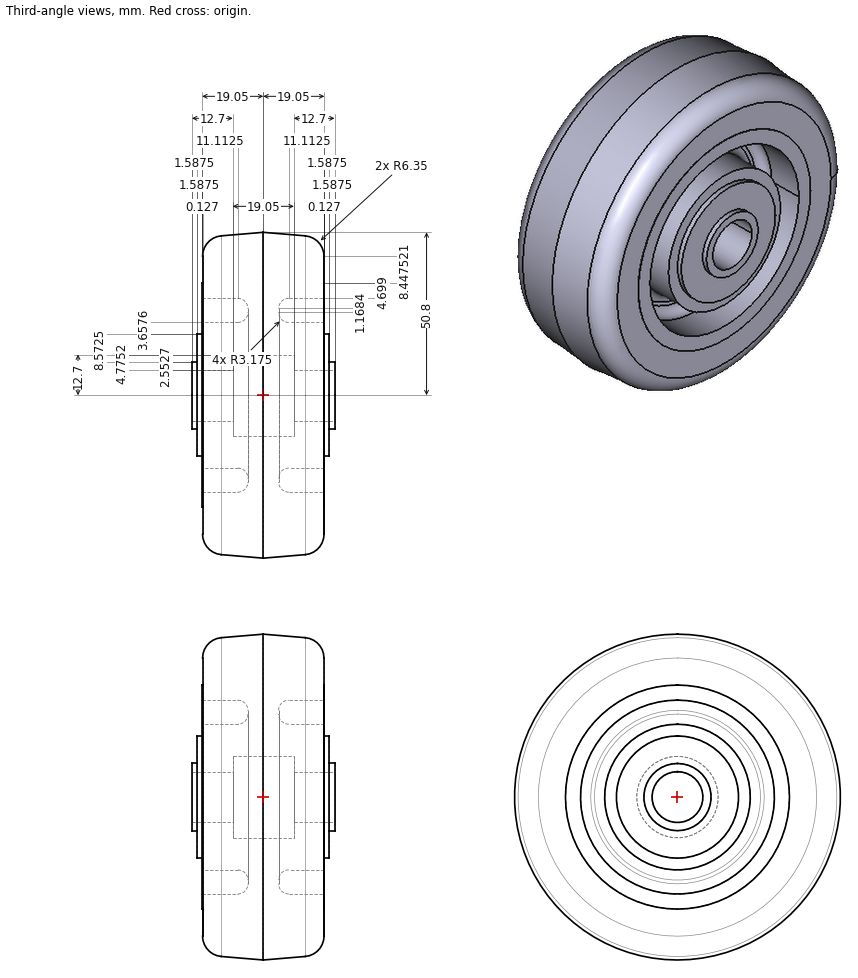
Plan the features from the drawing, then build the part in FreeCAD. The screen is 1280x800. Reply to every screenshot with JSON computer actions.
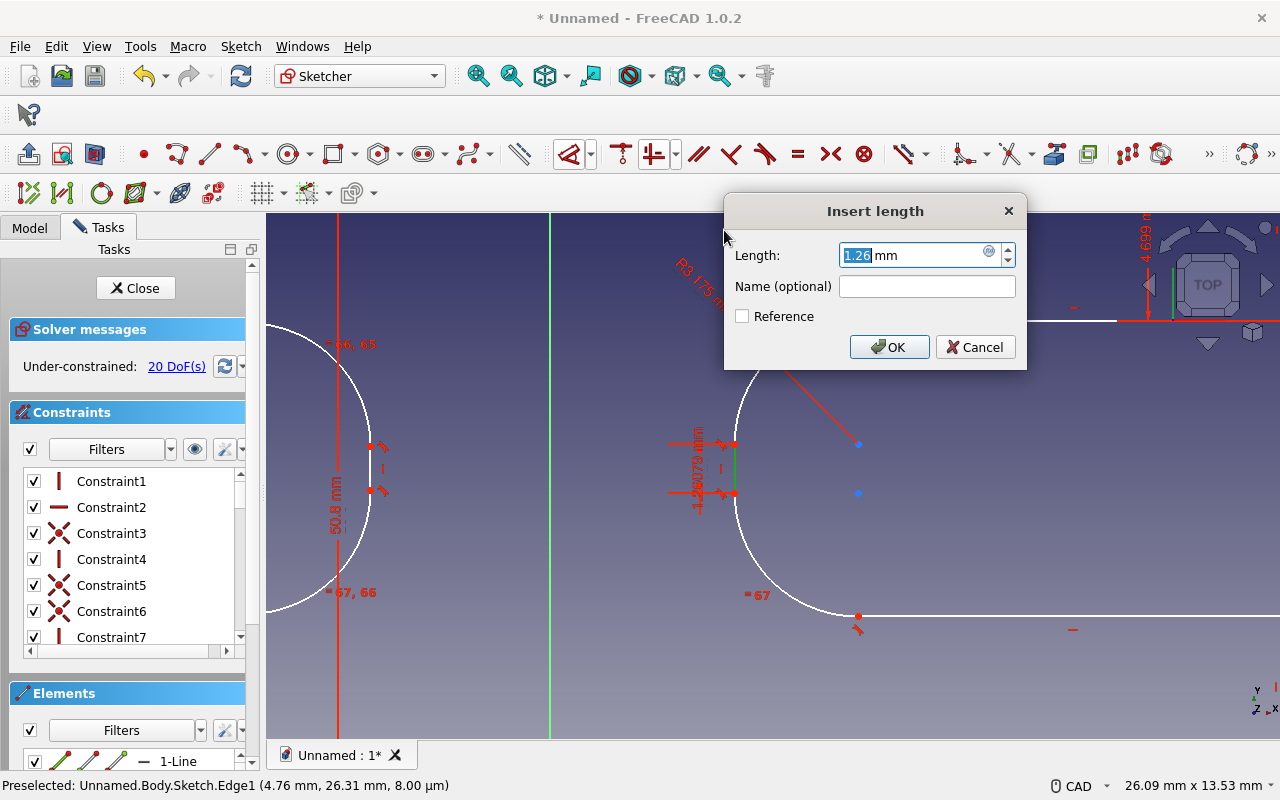
{"action": "type", "text": "1.1684"}
{"action": "key", "text": "Return"}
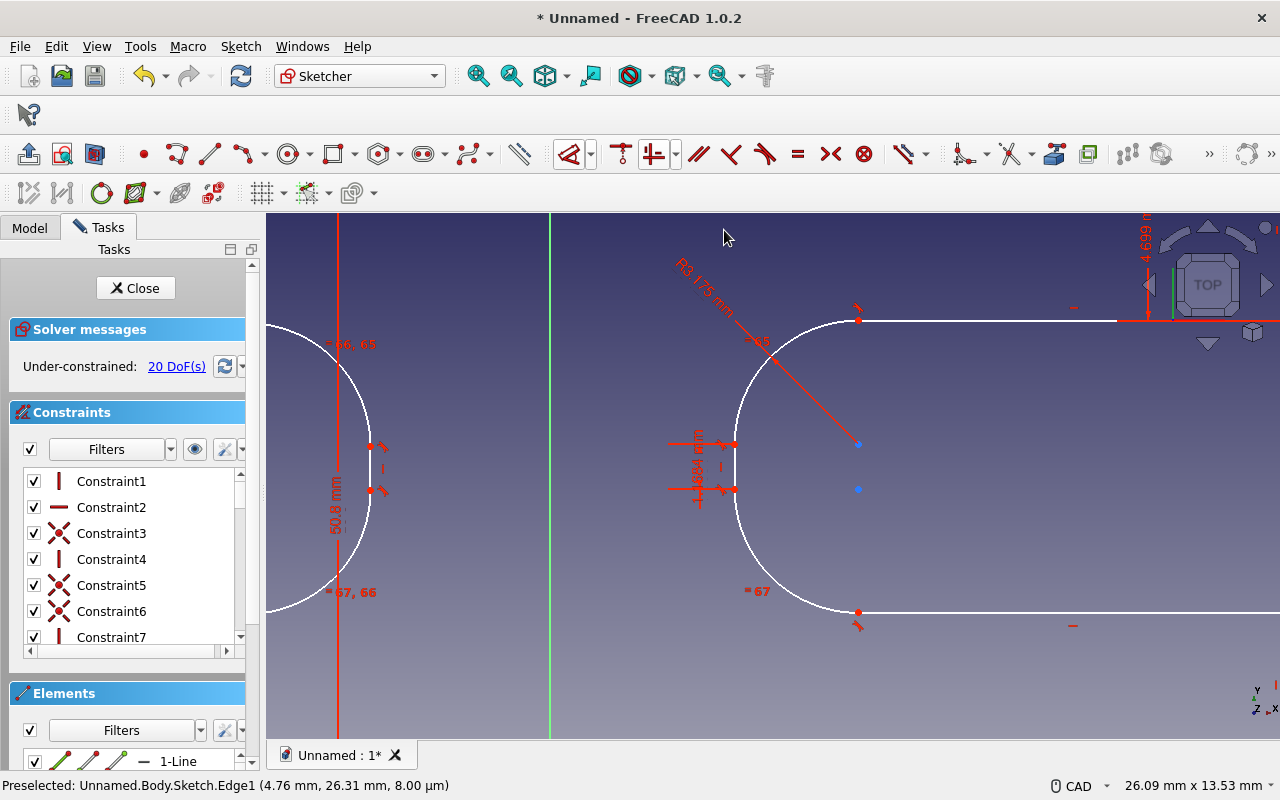
{"action": "left_click", "coordinate": [370, 460]}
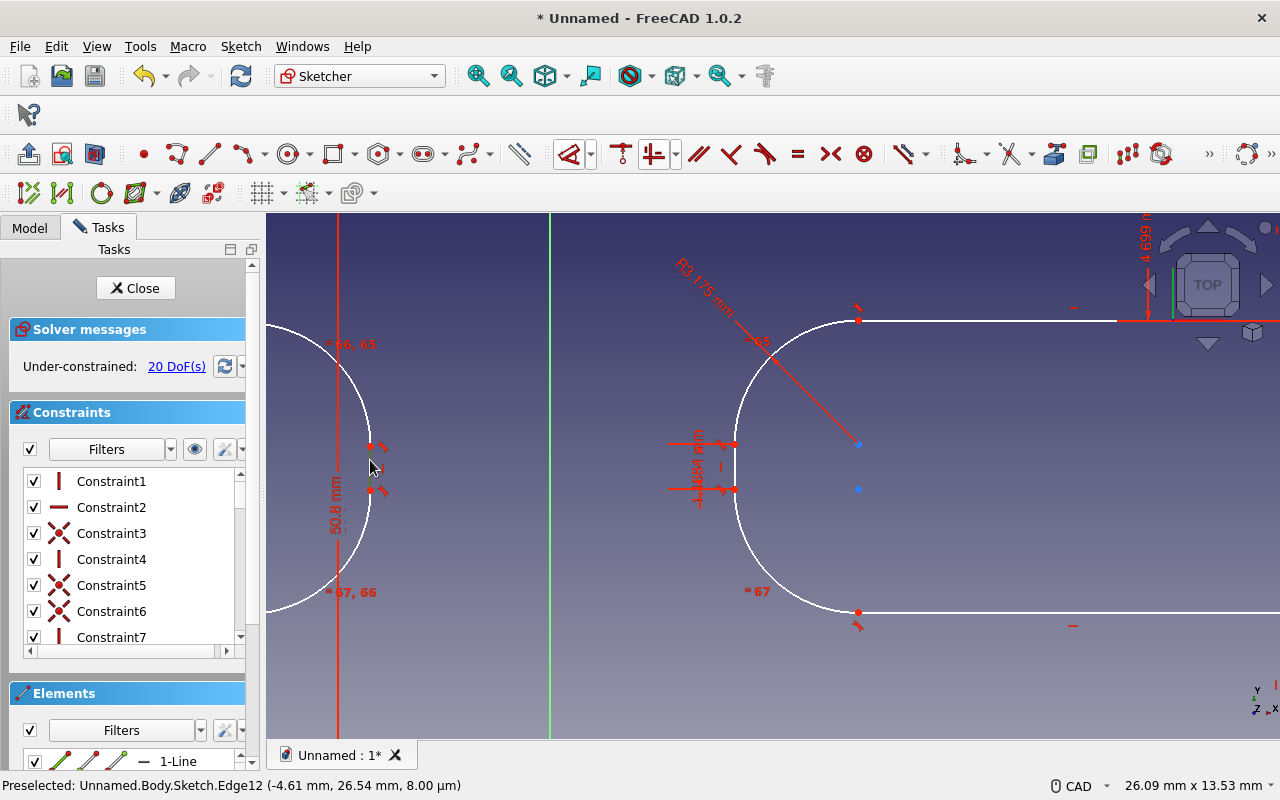
{"action": "left_click", "coordinate": [590, 154]}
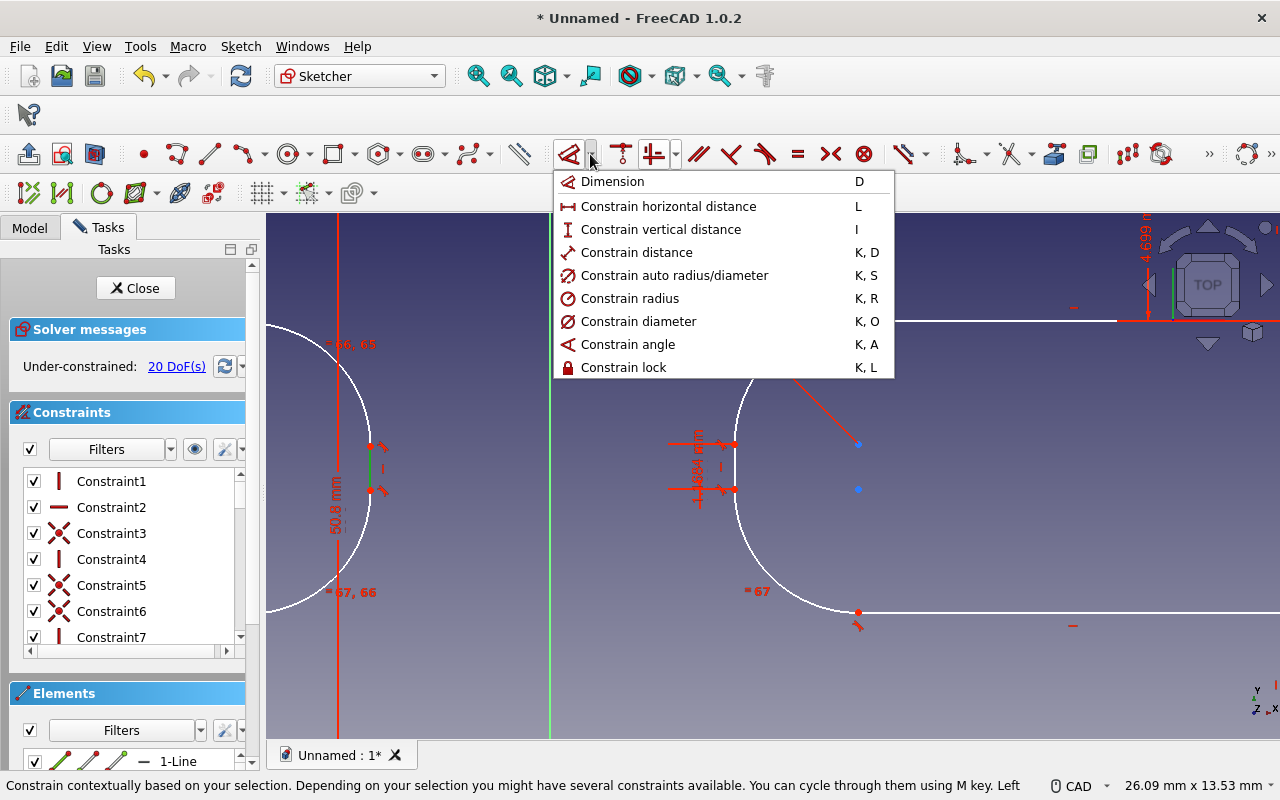
{"action": "left_click", "coordinate": [724, 230]}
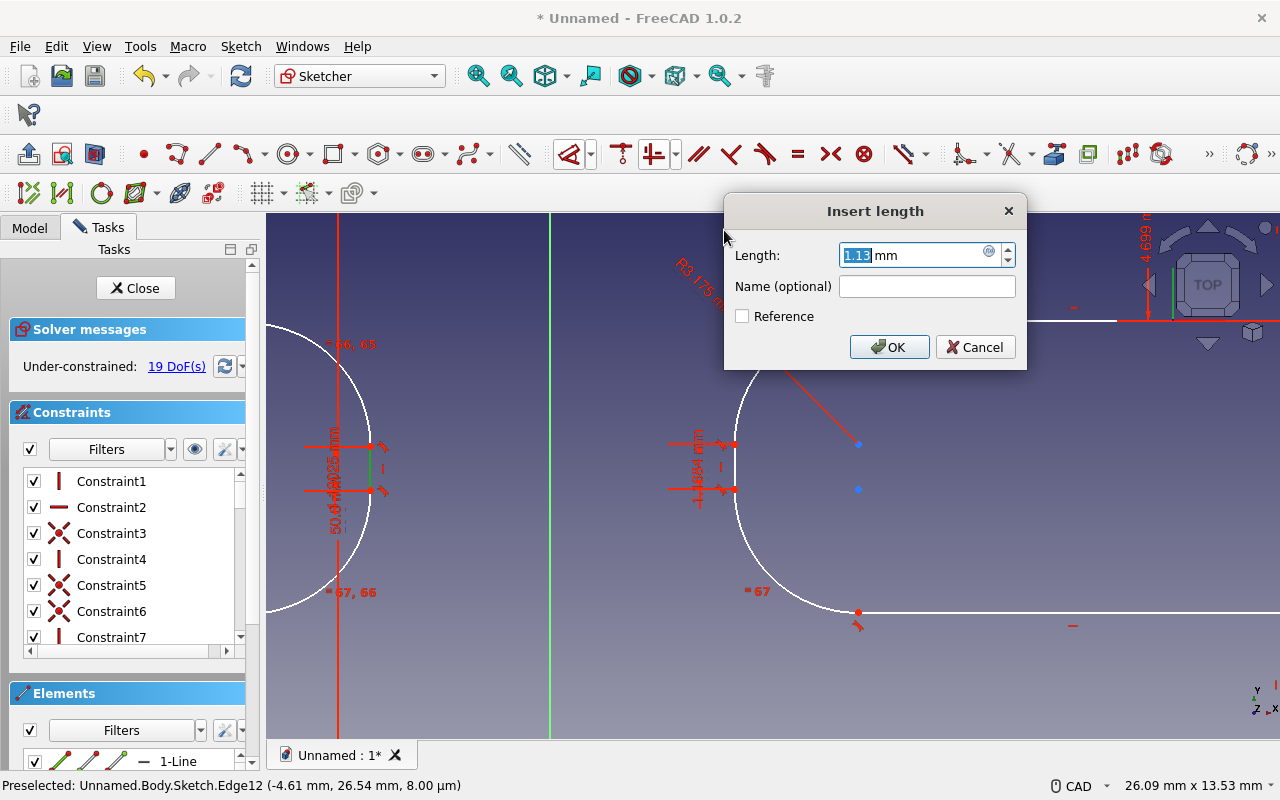
{"action": "type", "text": "1.1684"}
{"action": "key", "text": "Return"}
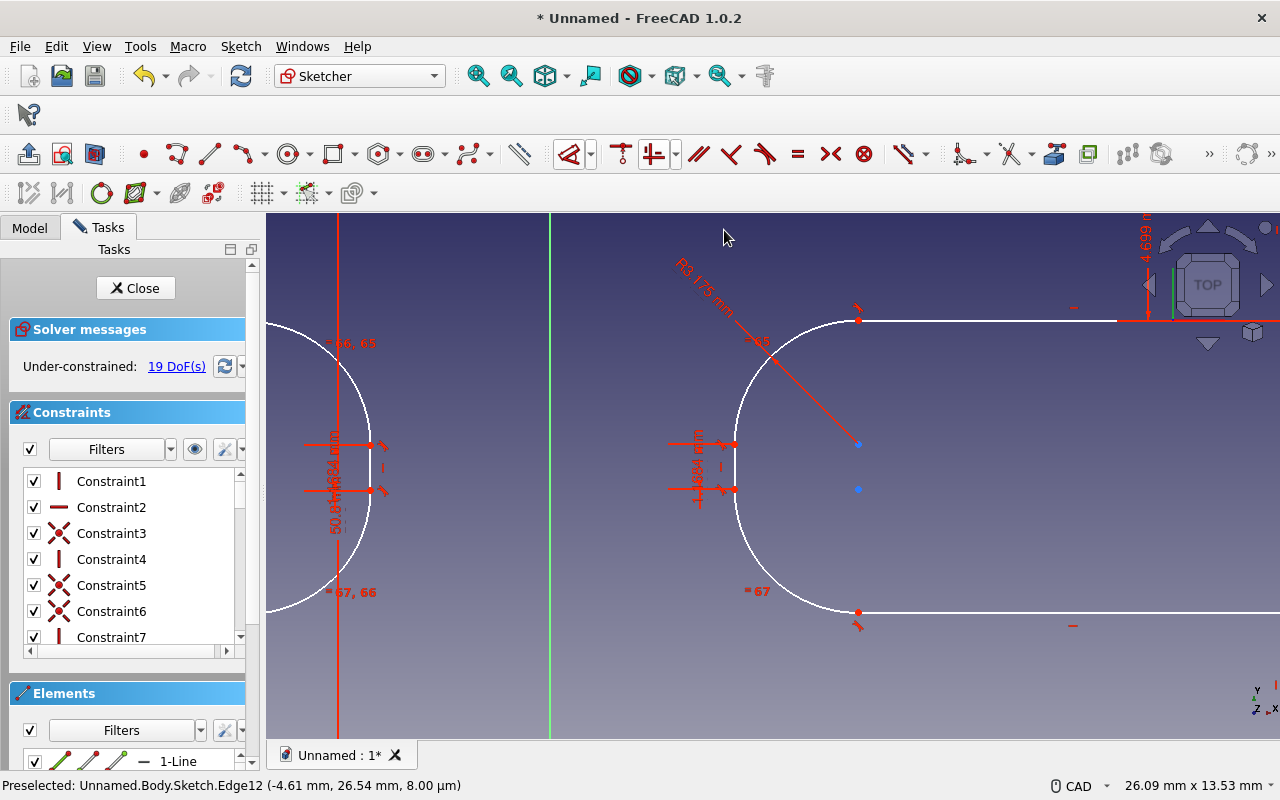
{"action": "scroll", "coordinate": [735, 470], "scroll_direction": "down", "scroll_amount": 9}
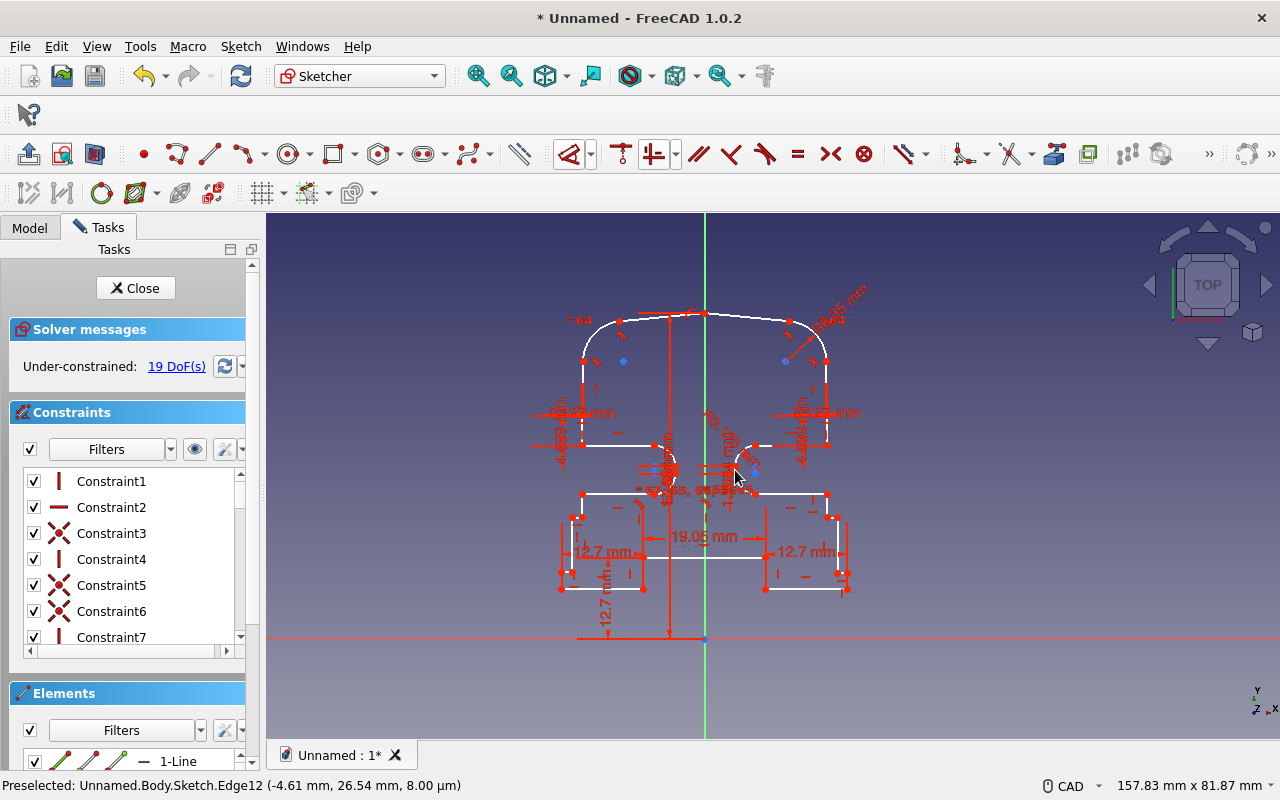
{"action": "scroll", "coordinate": [582, 501], "scroll_direction": "up", "scroll_amount": 4}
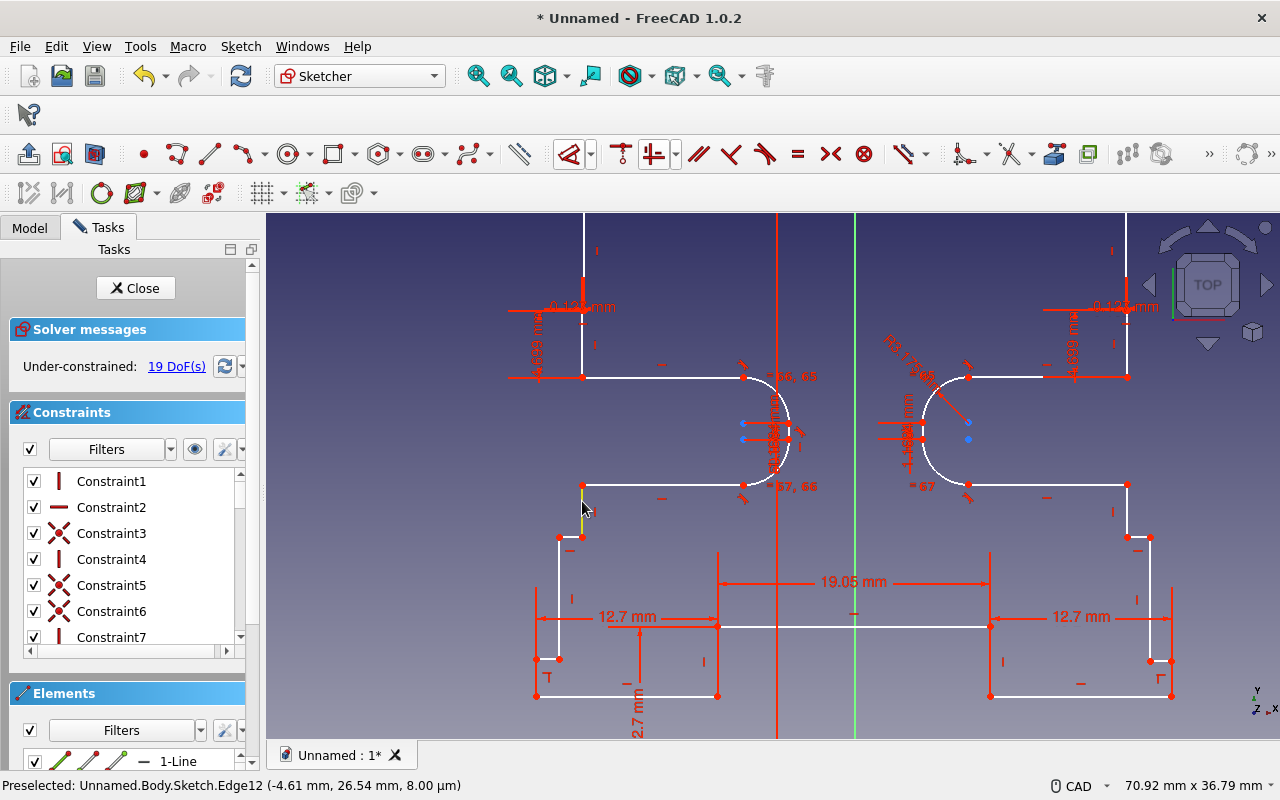
{"action": "left_click", "coordinate": [582, 501]}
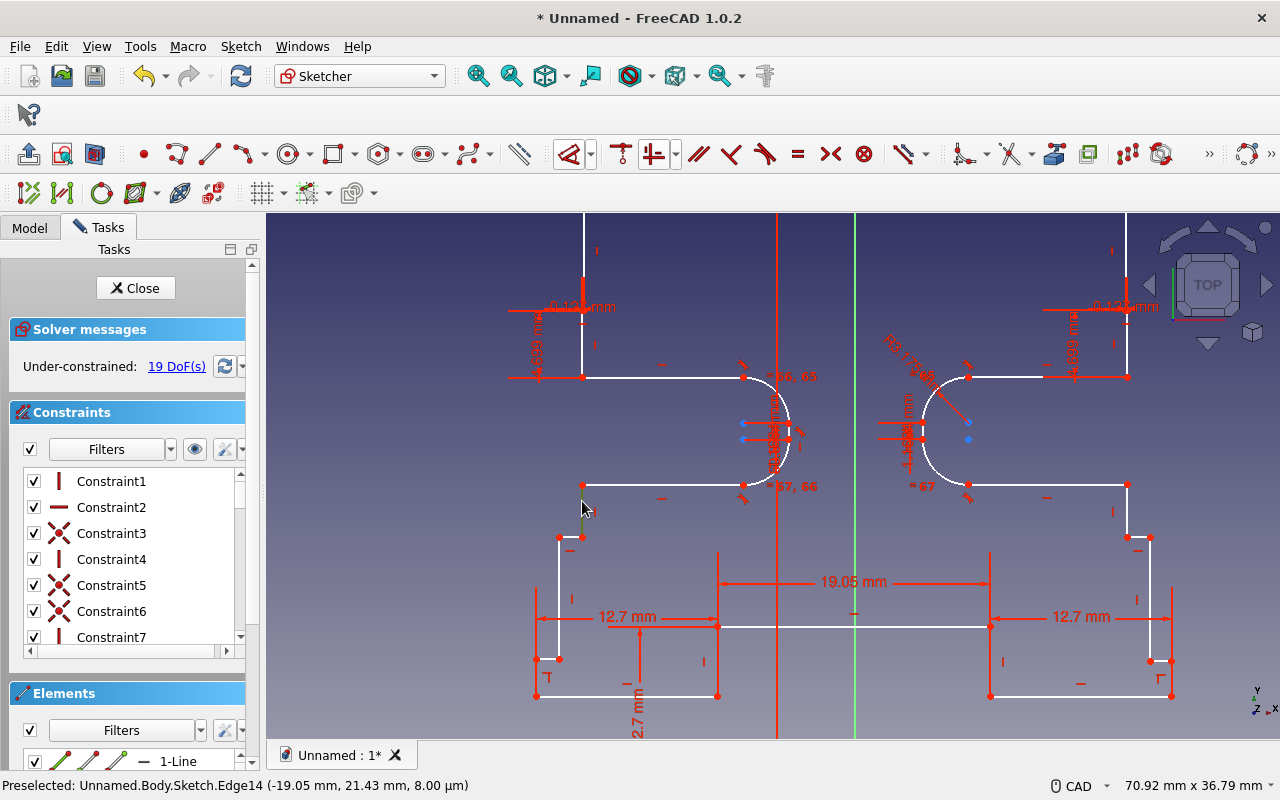
{"action": "key", "text": "i"}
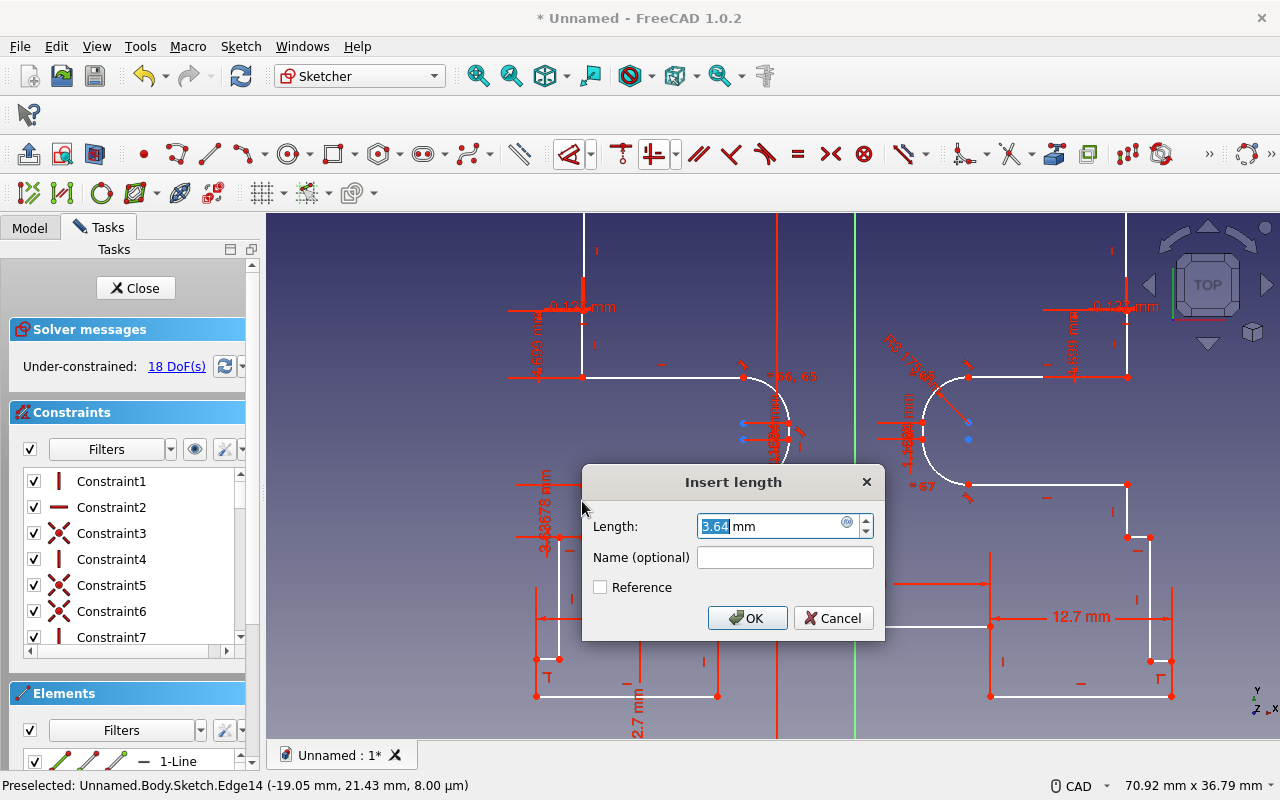
{"action": "type", "text": "3.6576"}
{"action": "key", "text": "Return"}